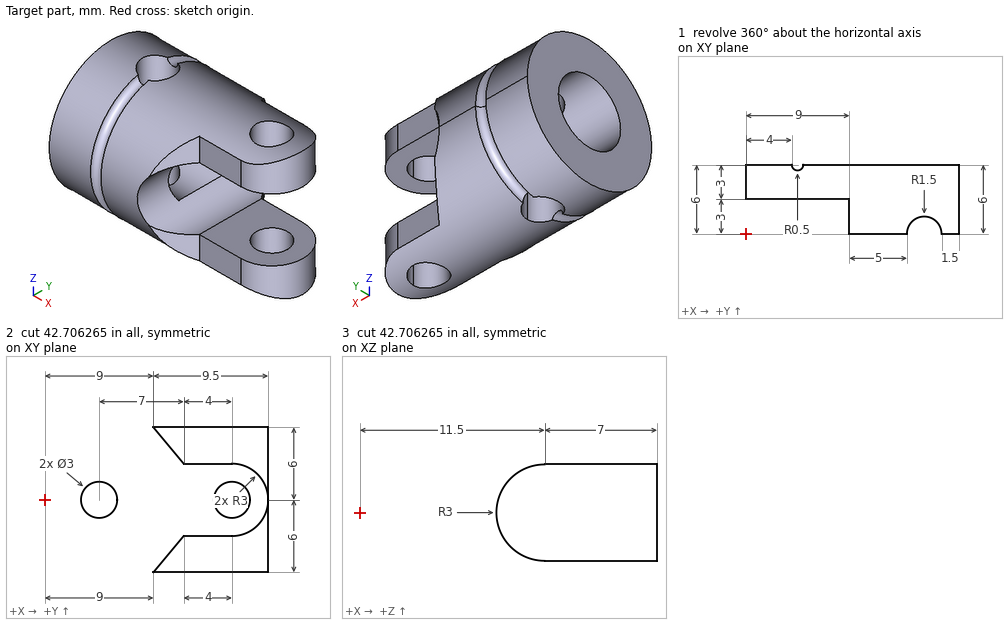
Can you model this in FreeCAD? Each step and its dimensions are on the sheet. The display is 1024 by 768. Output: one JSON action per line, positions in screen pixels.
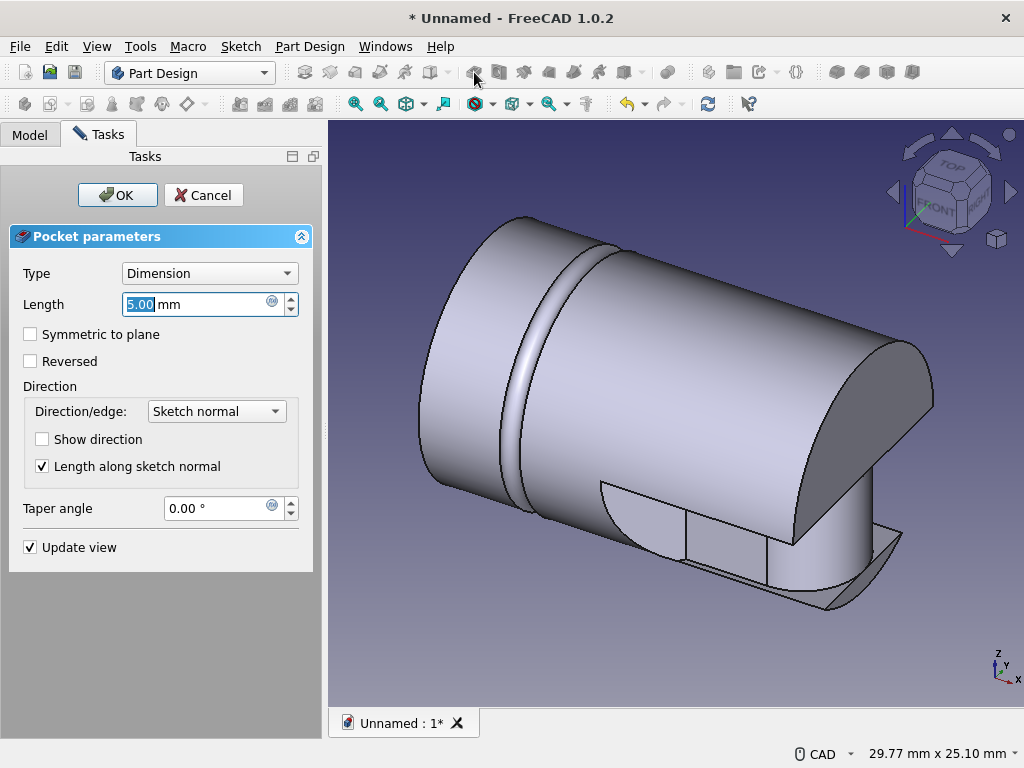
{"action": "type", "text": "42.706265"}
{"action": "key", "text": "Tab"}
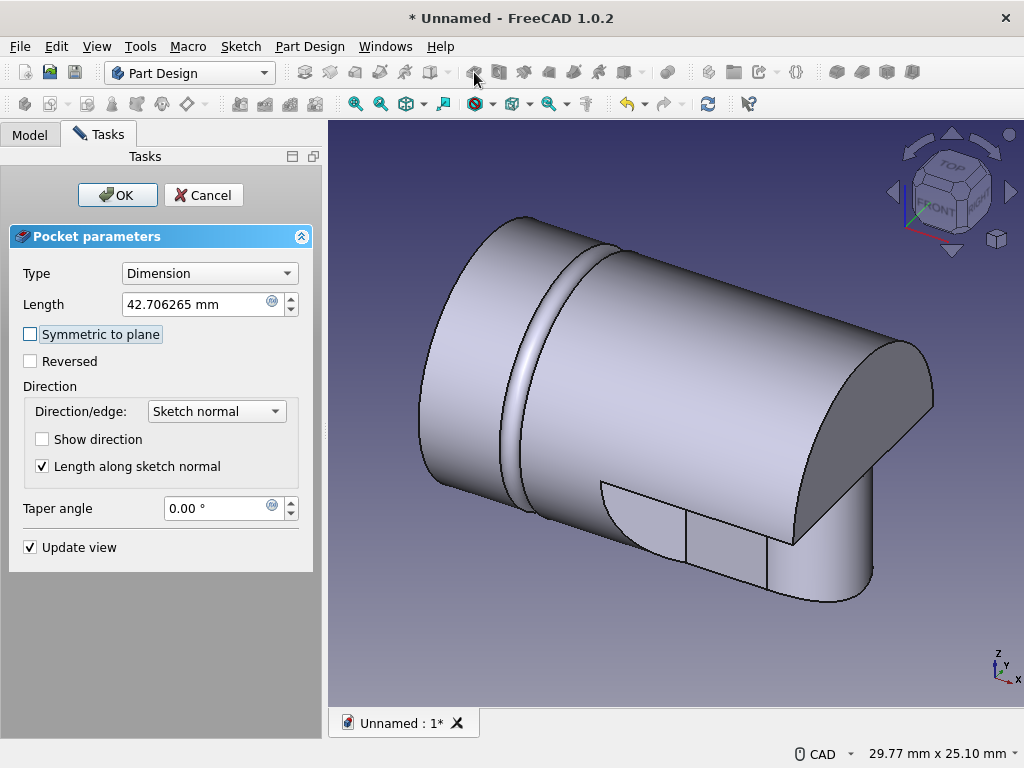
{"action": "left_click", "coordinate": [31, 334]}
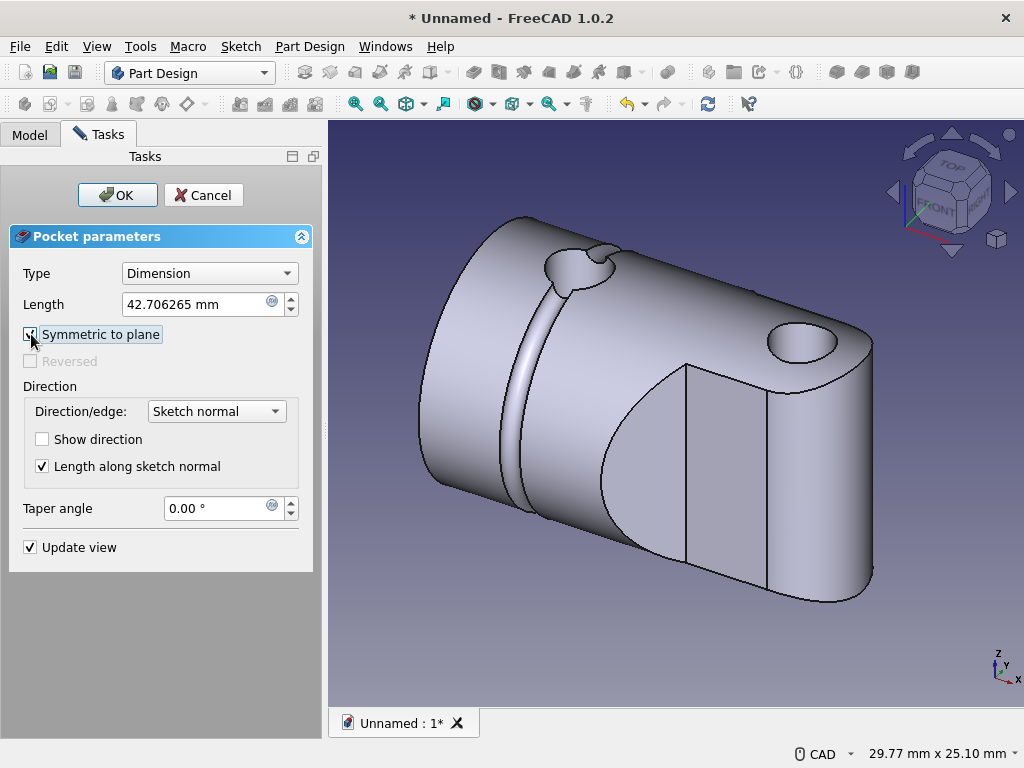
{"action": "left_click", "coordinate": [118, 195]}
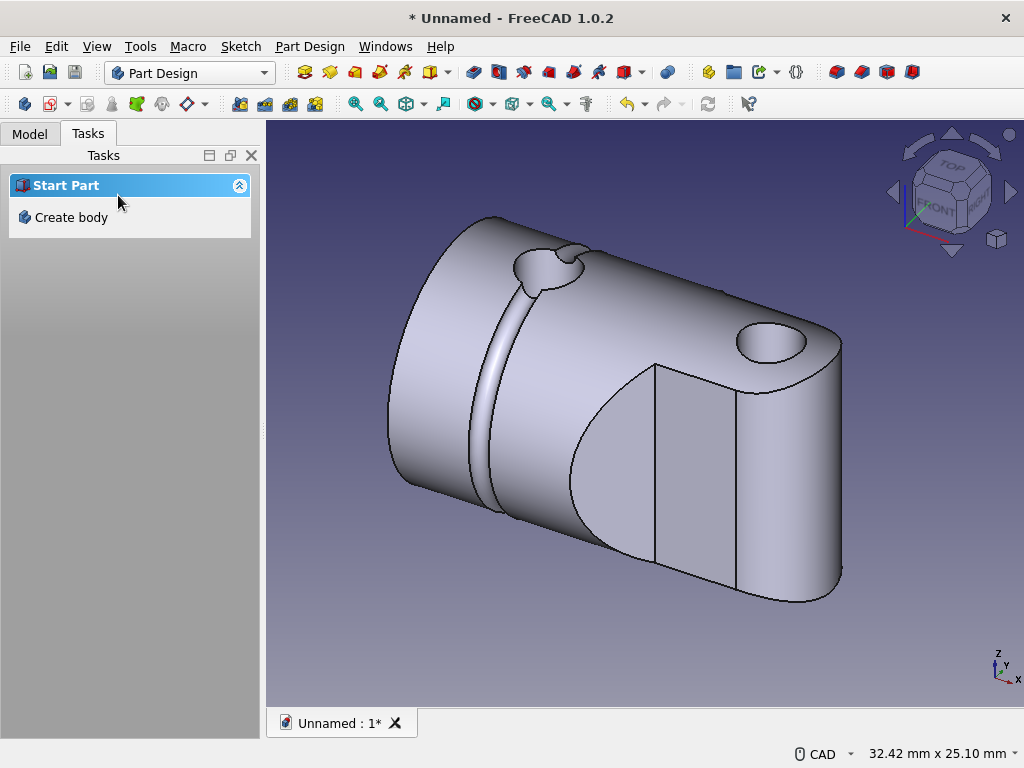
{"action": "left_click", "coordinate": [50, 104]}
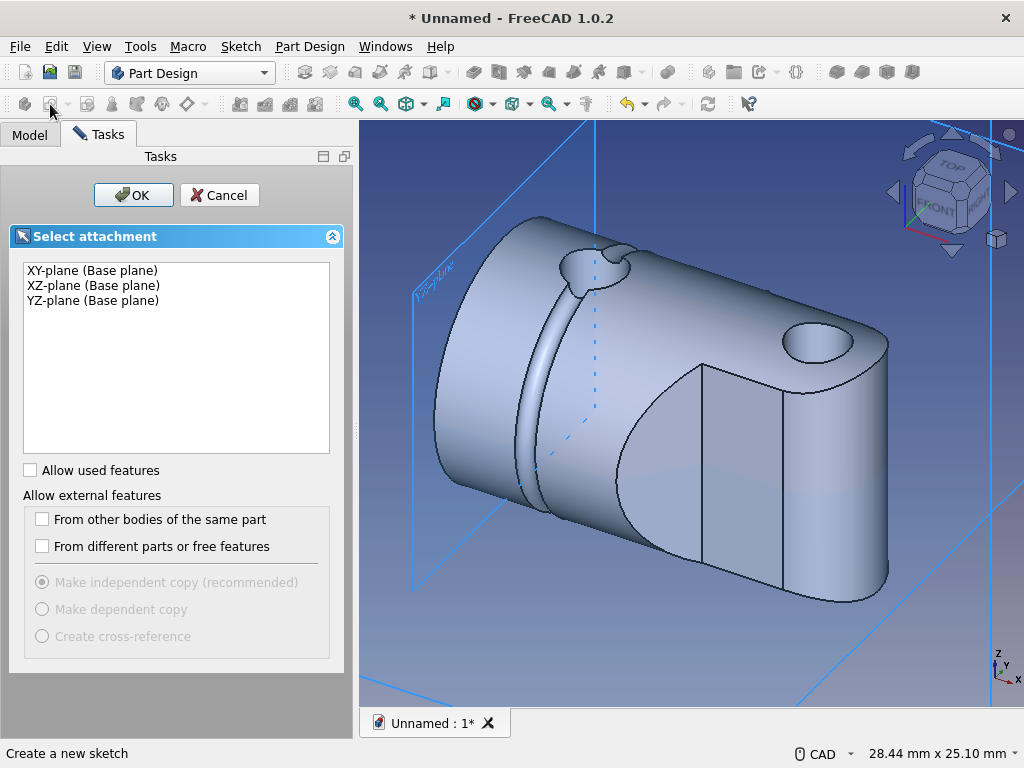
{"action": "left_click", "coordinate": [84, 286]}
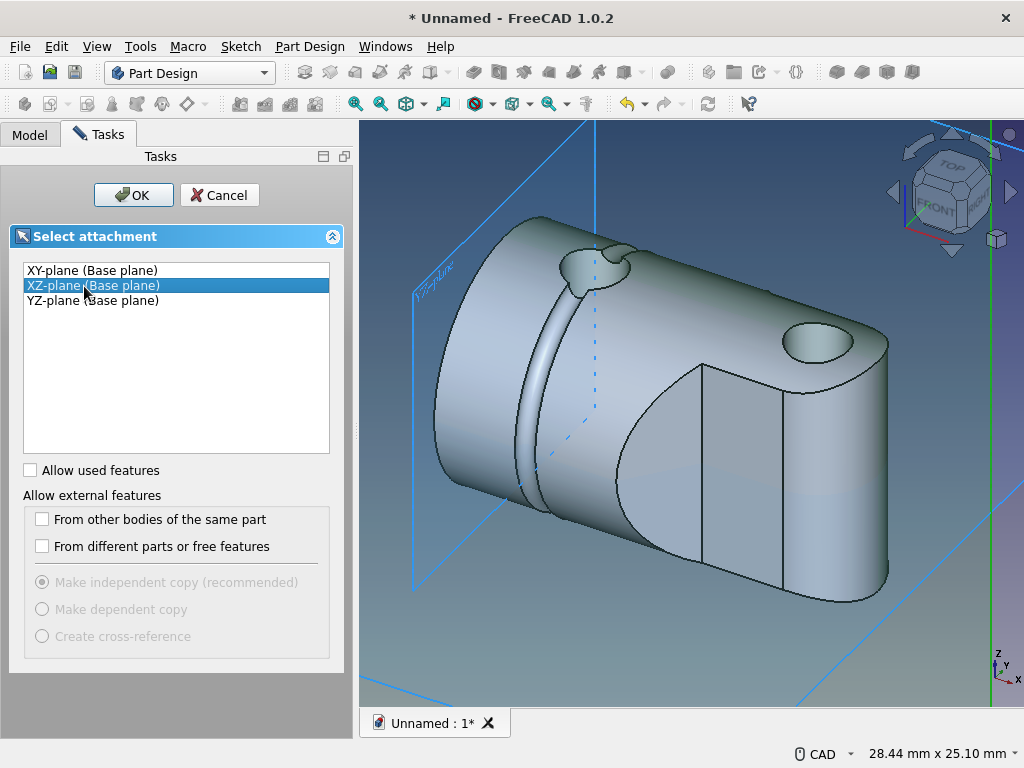
{"action": "left_click", "coordinate": [134, 195]}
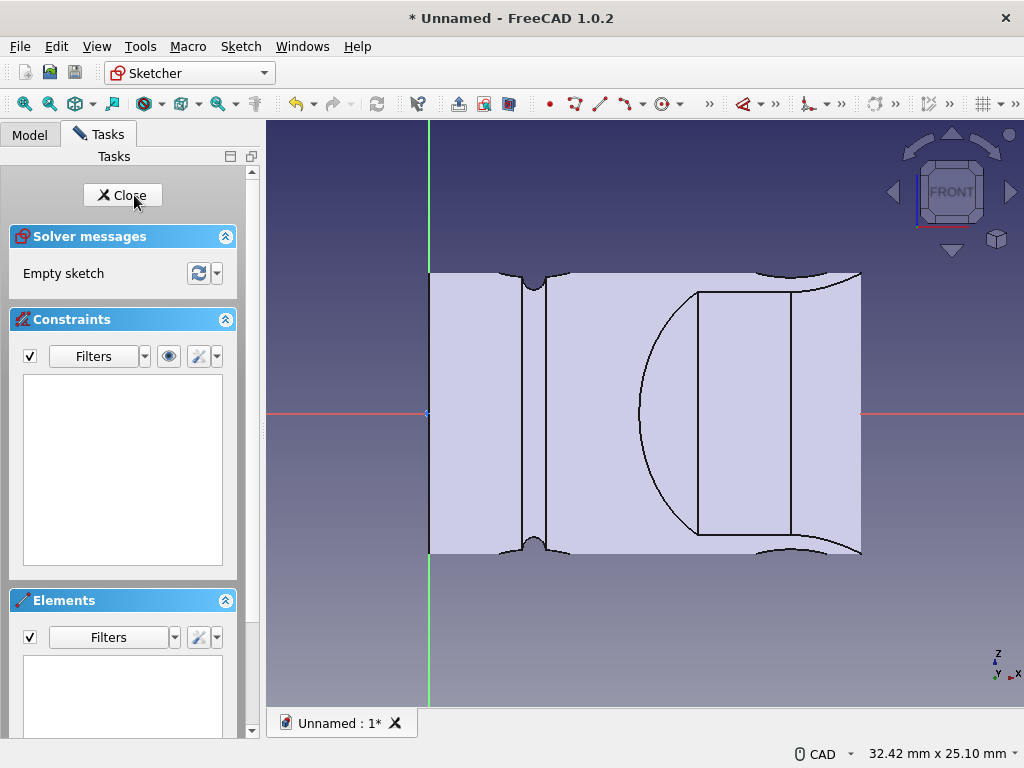
{"action": "left_click", "coordinate": [509, 104]}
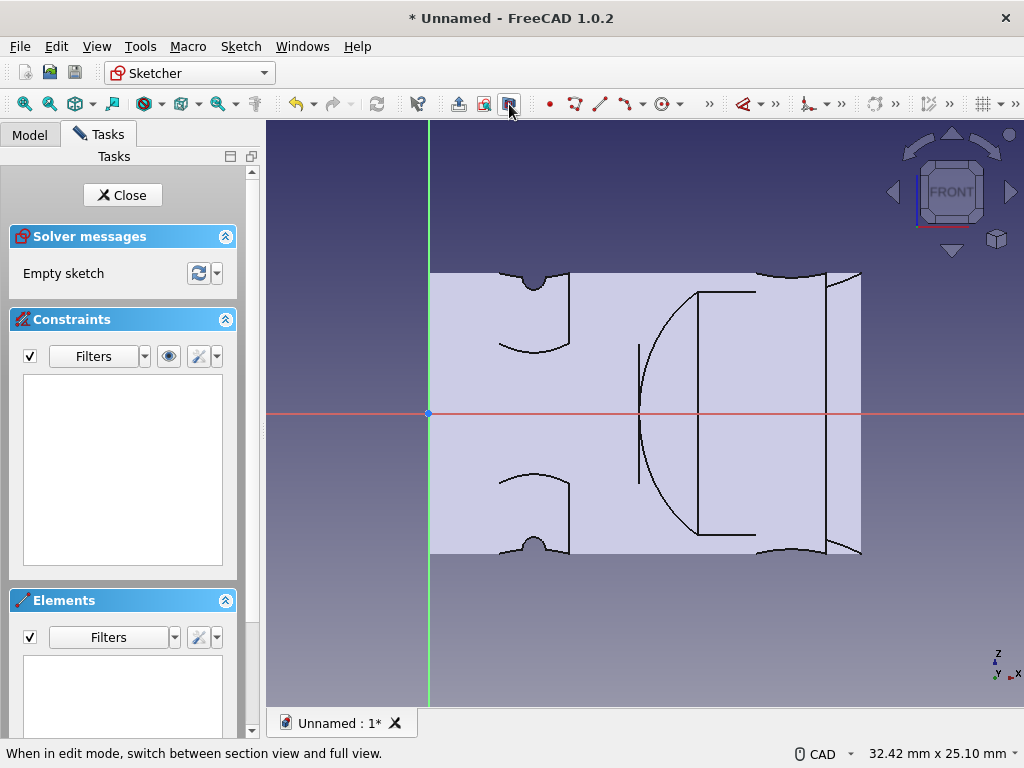
{"action": "scroll", "coordinate": [294, 413], "scroll_direction": "down", "scroll_amount": 1}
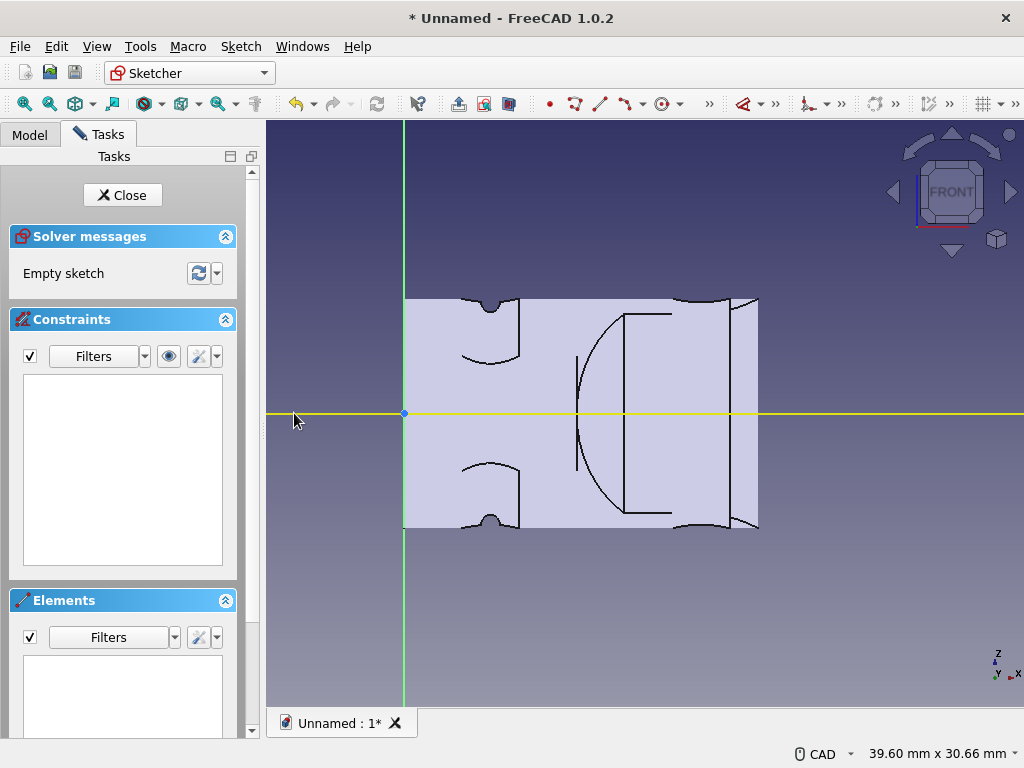
{"action": "key", "text": "g m"}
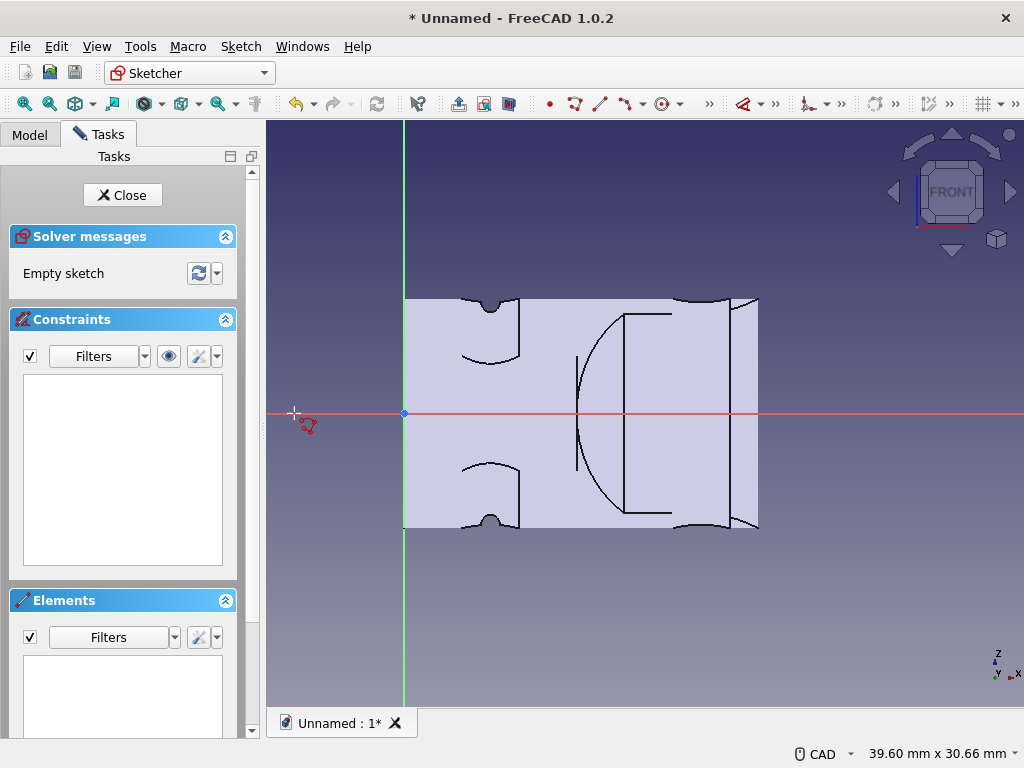
{"action": "left_click", "coordinate": [624, 356]}
{"action": "left_click", "coordinate": [758, 356]}
{"action": "left_click", "coordinate": [758, 471]}
{"action": "left_click", "coordinate": [624, 471]}
{"action": "right_click", "coordinate": [624, 471]}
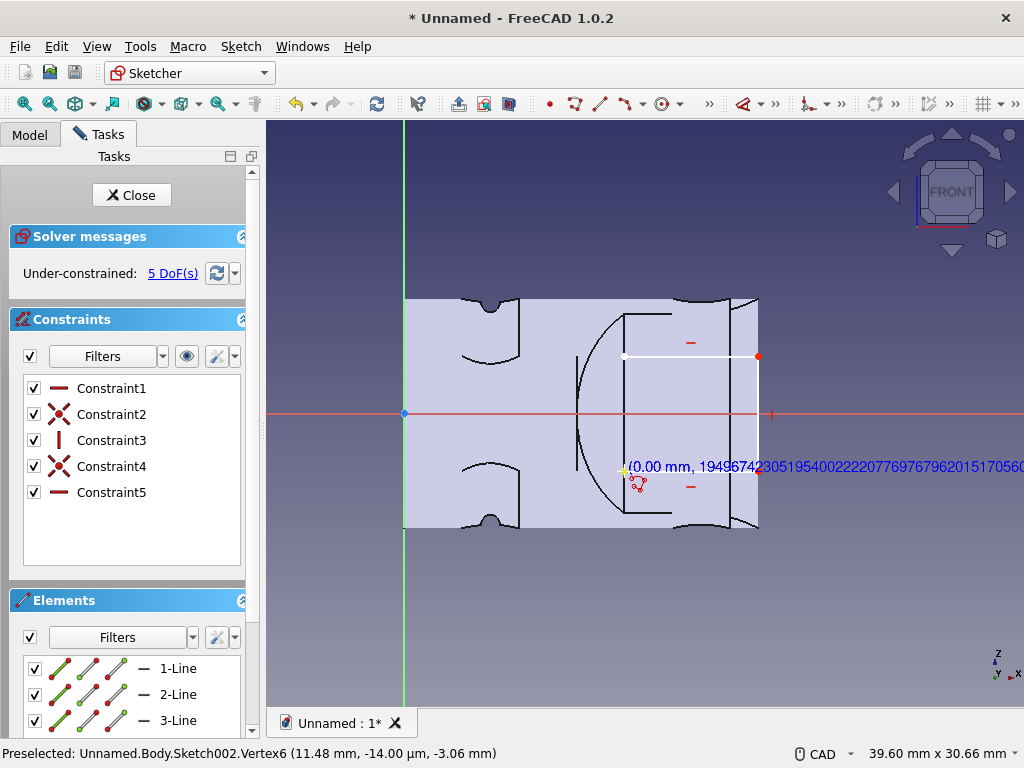
{"action": "key", "text": "g 3 a"}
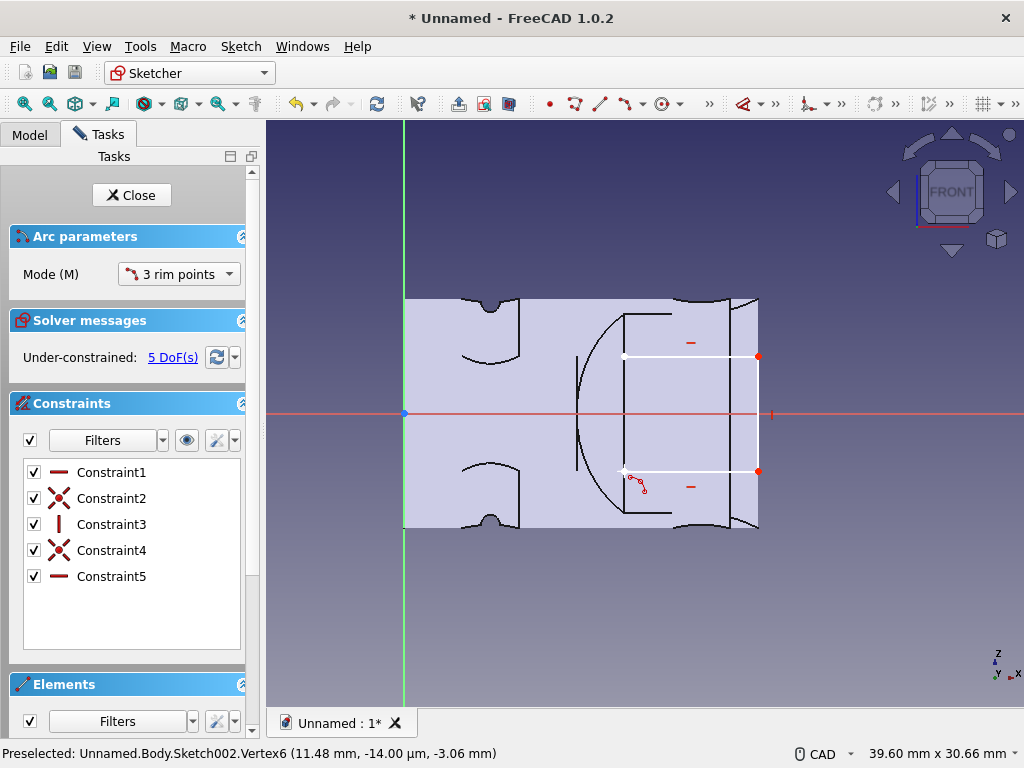
{"action": "left_click", "coordinate": [624, 472]}
{"action": "left_click", "coordinate": [624, 357]}
{"action": "left_click", "coordinate": [570, 396]}
{"action": "key", "text": "Escape"}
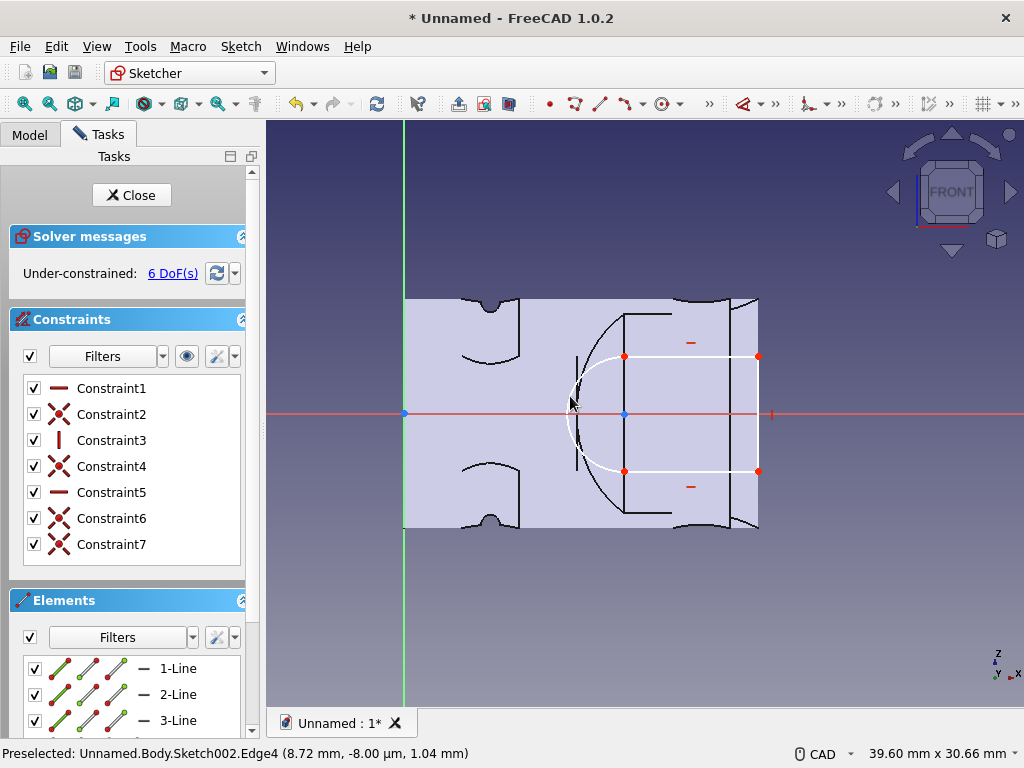
{"action": "left_click", "coordinate": [664, 357]}